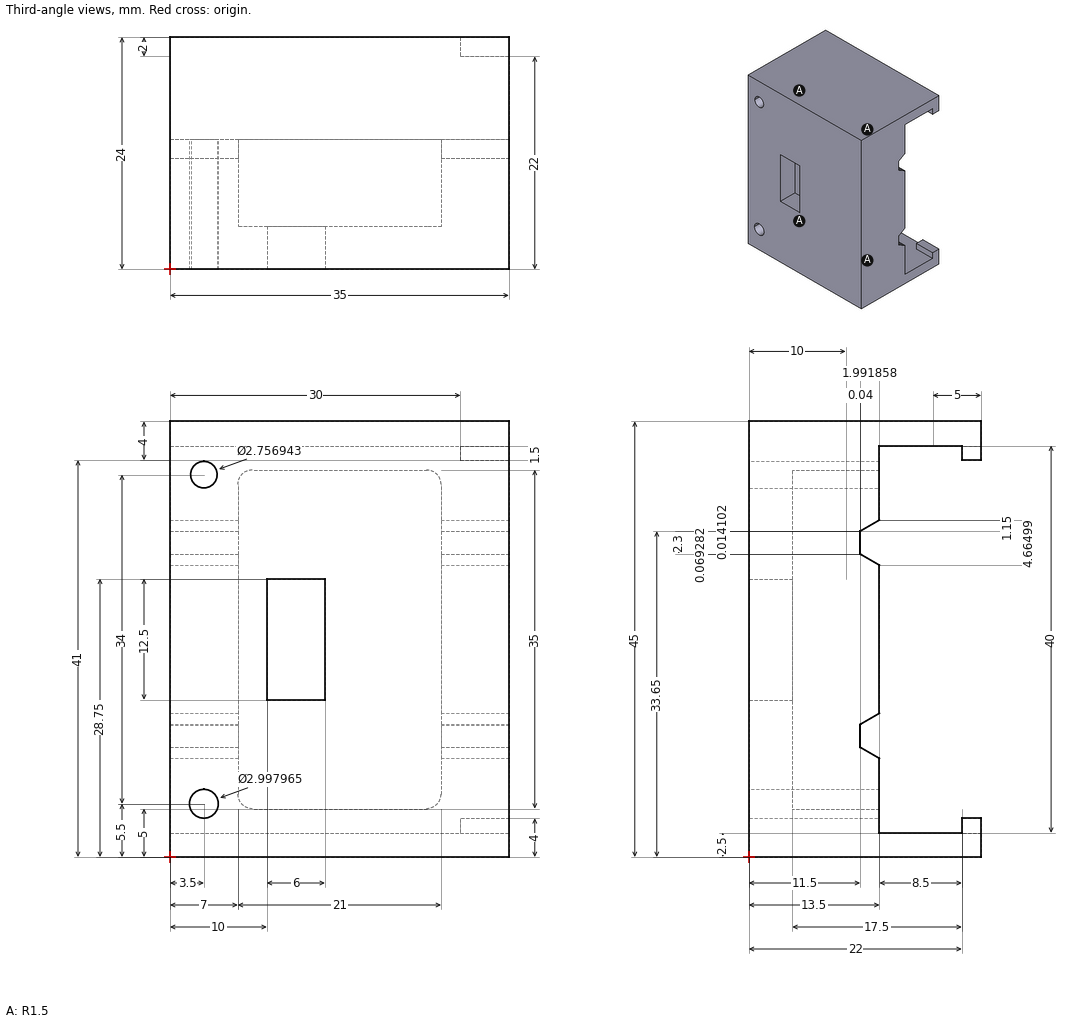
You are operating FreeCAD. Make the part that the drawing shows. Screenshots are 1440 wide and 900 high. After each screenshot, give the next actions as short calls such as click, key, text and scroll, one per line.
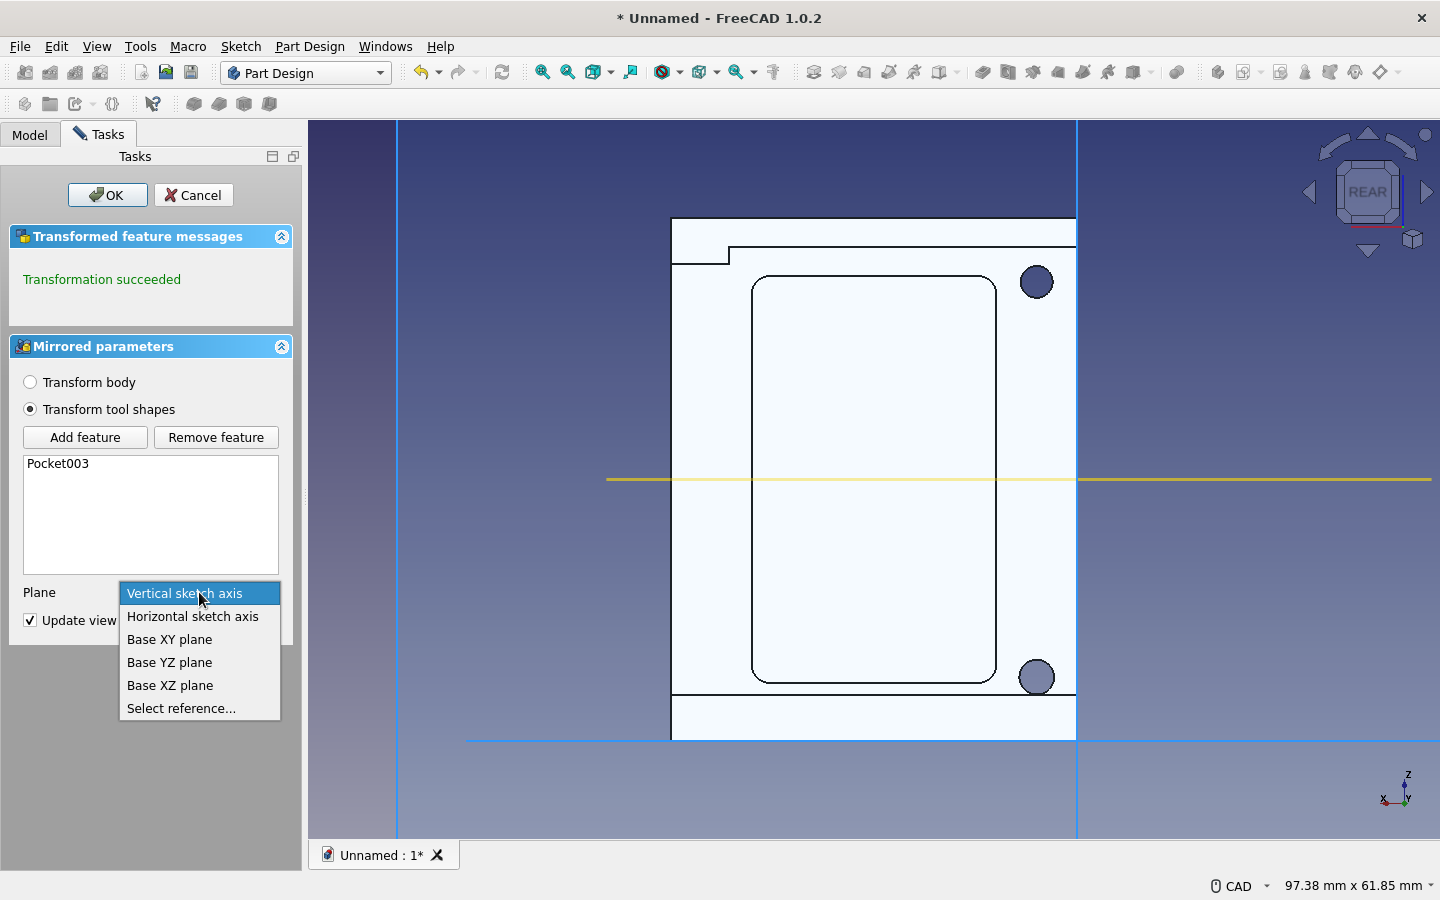
click(198, 708)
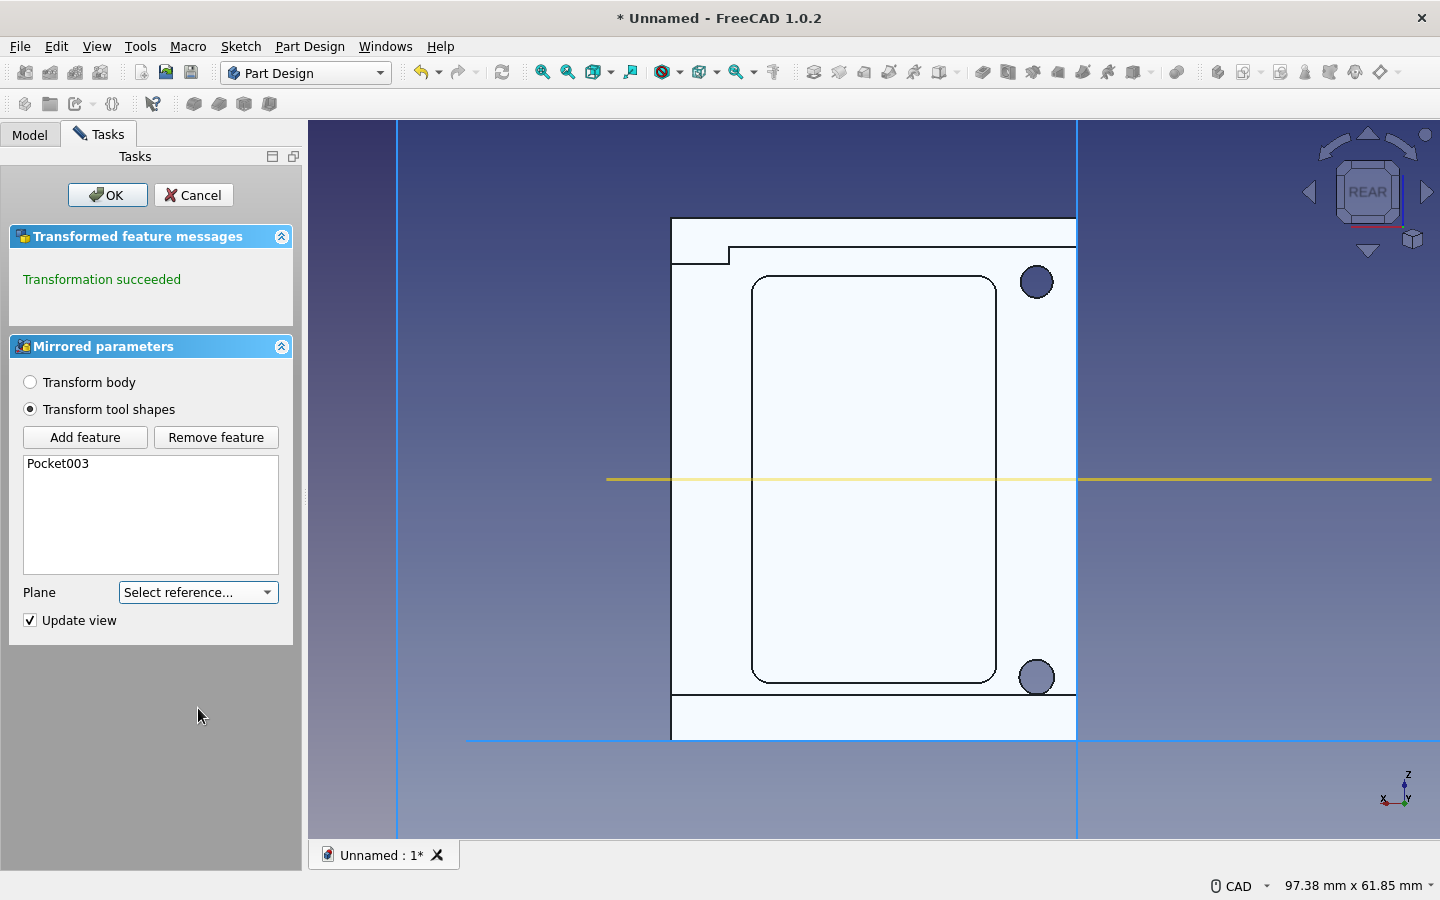
click(30, 134)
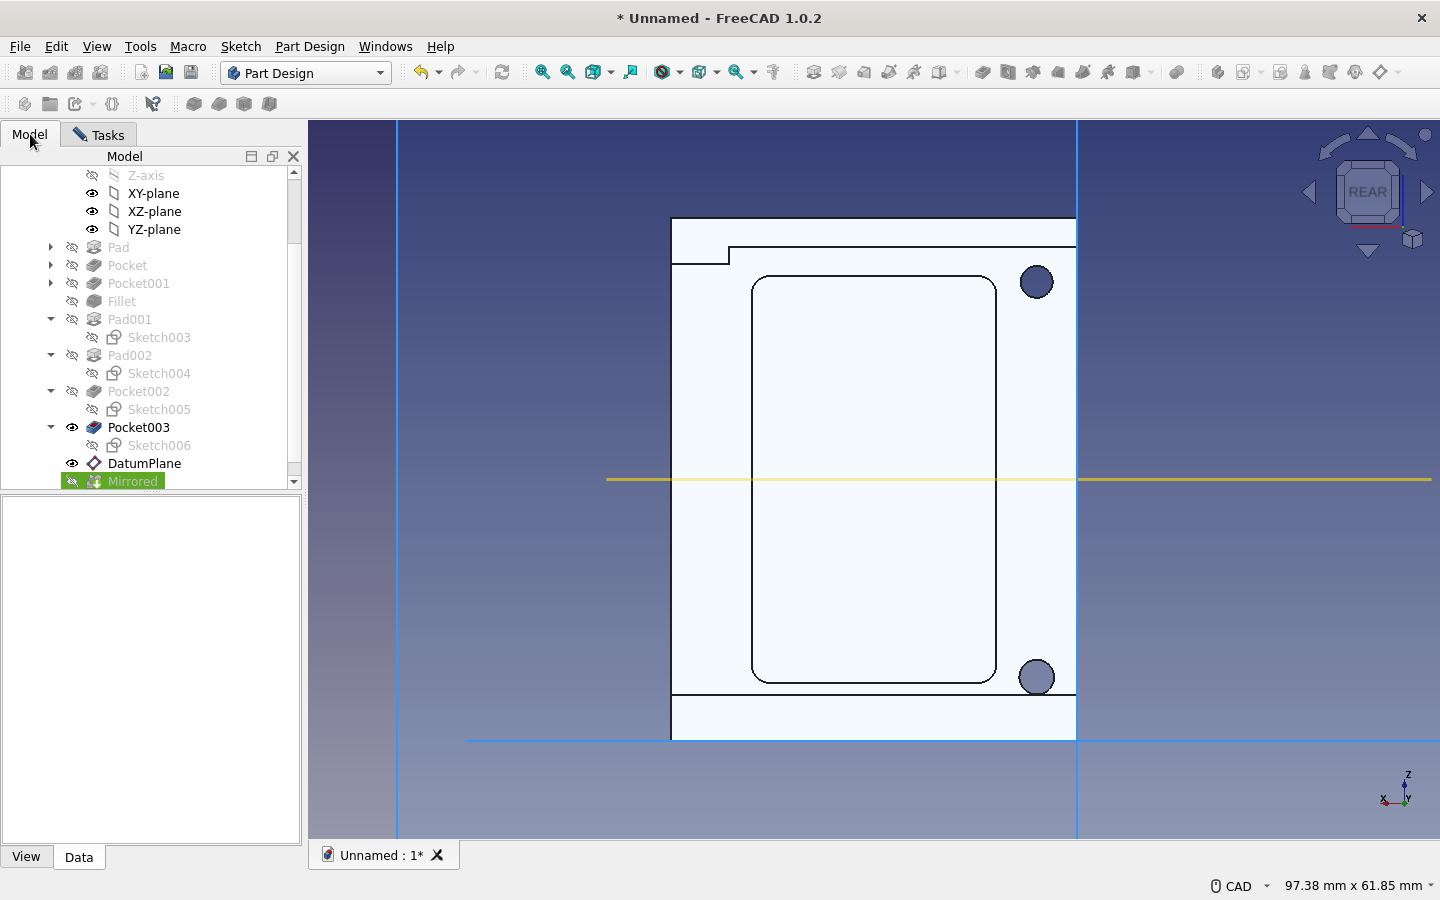
click(117, 463)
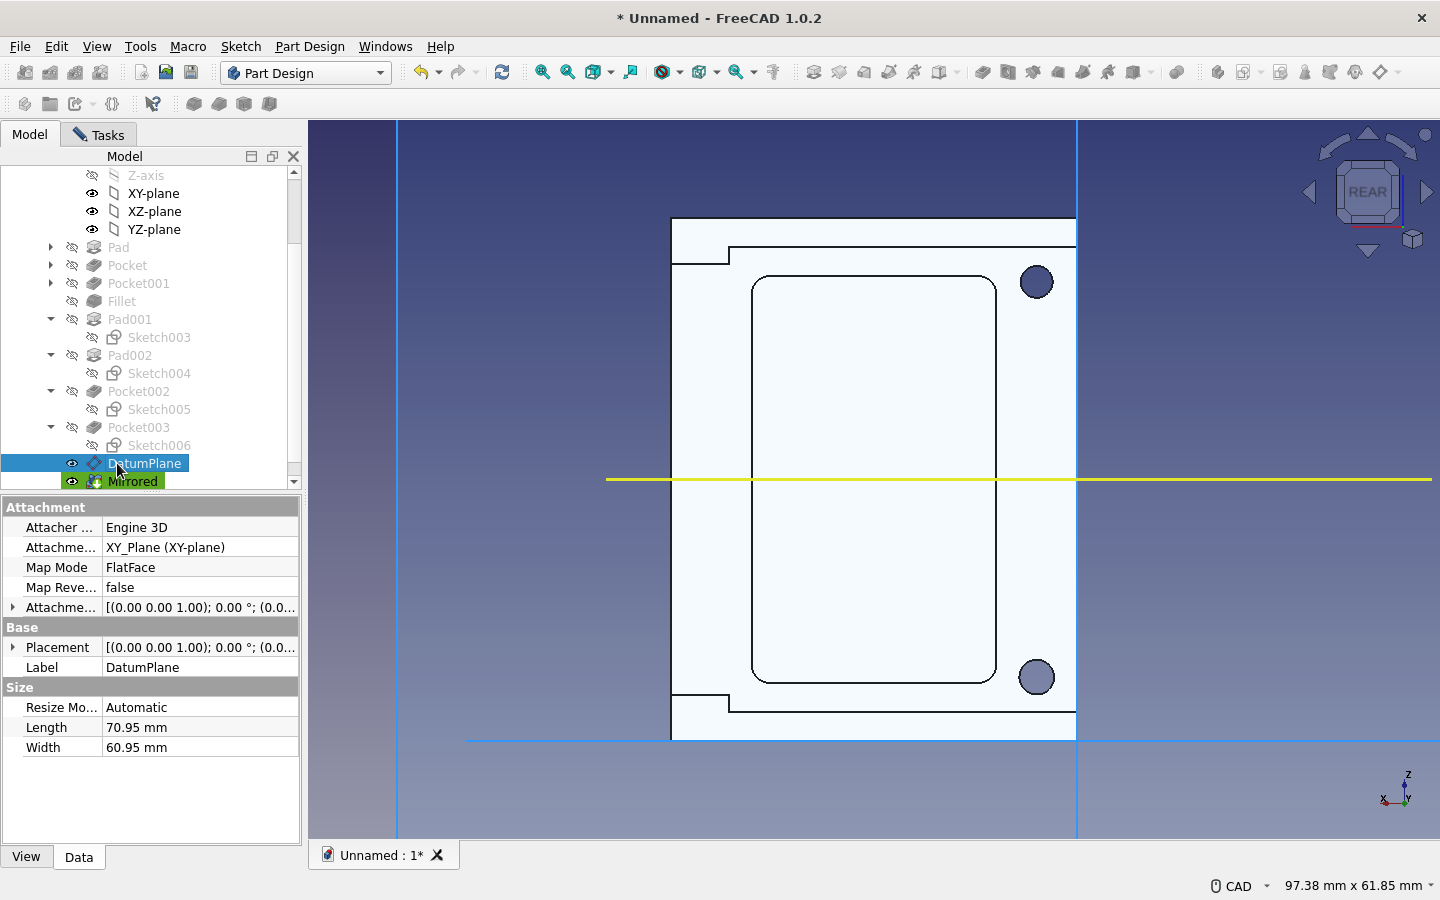
click(98, 134)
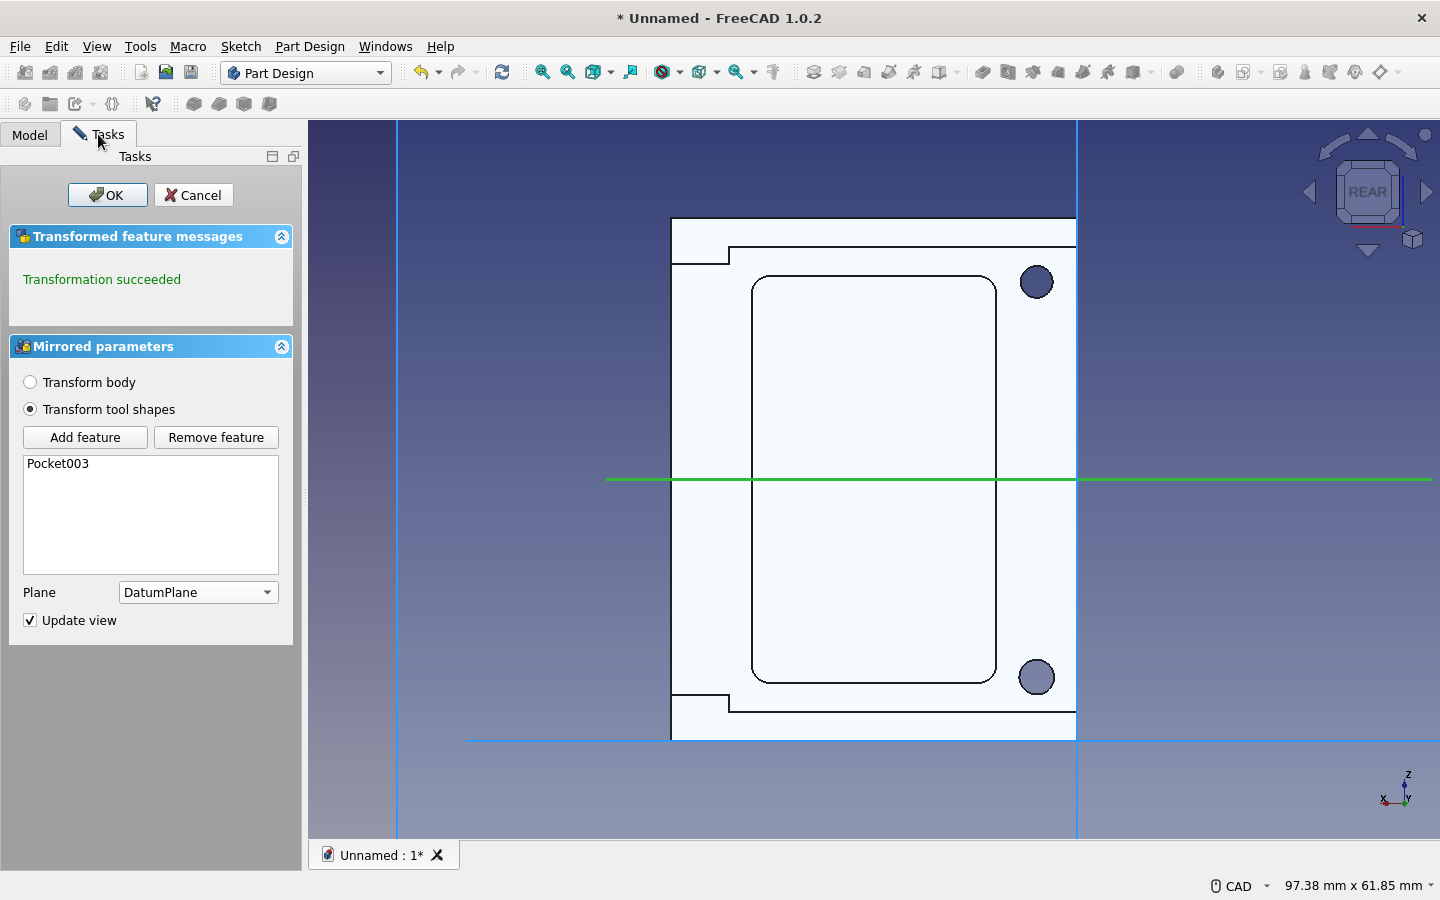
click(108, 195)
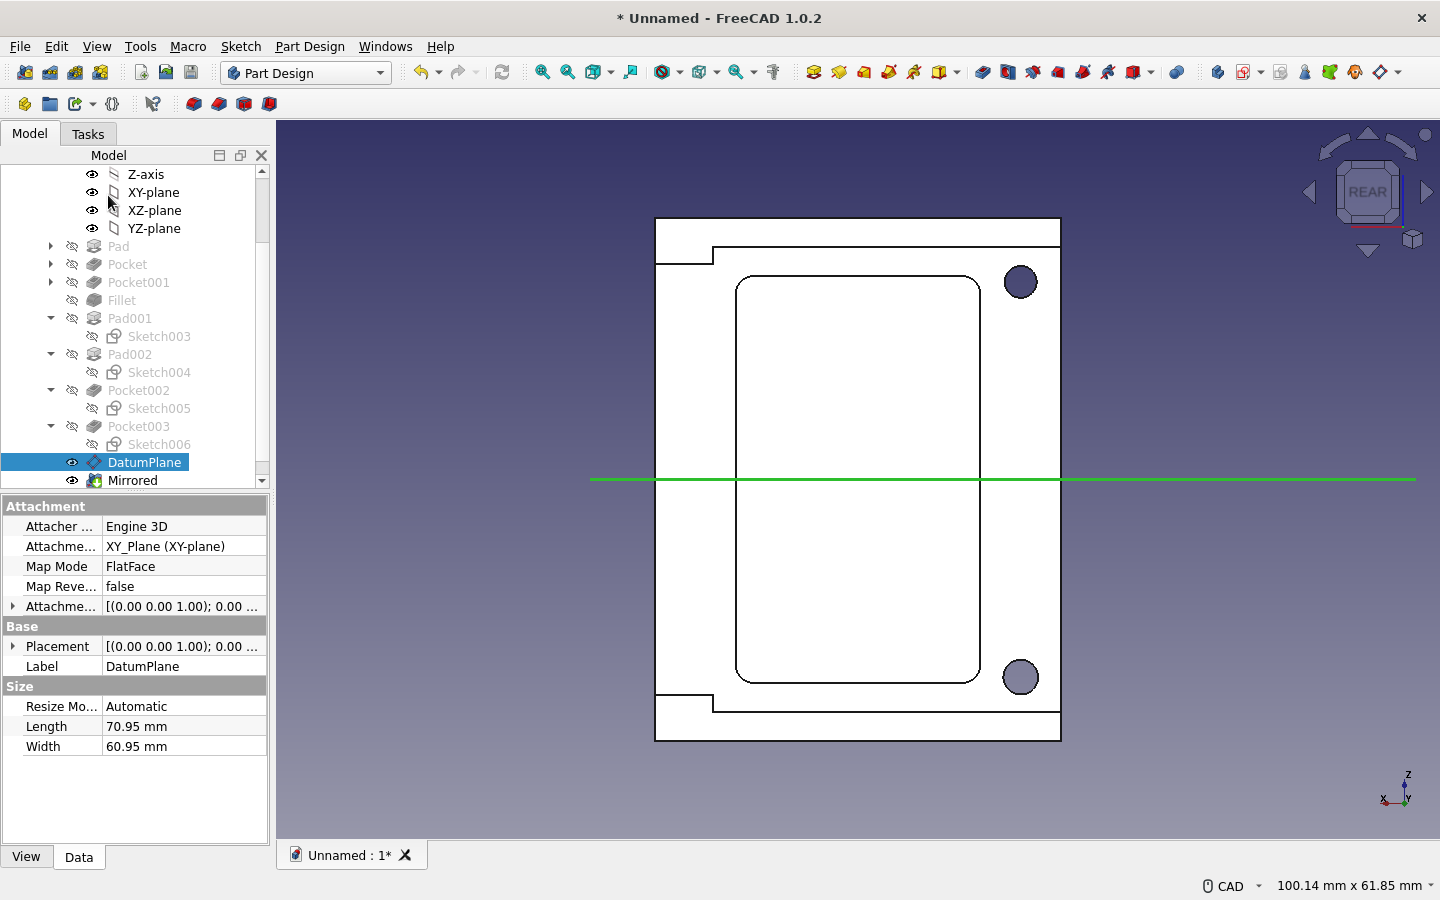
click(117, 462)
key(space)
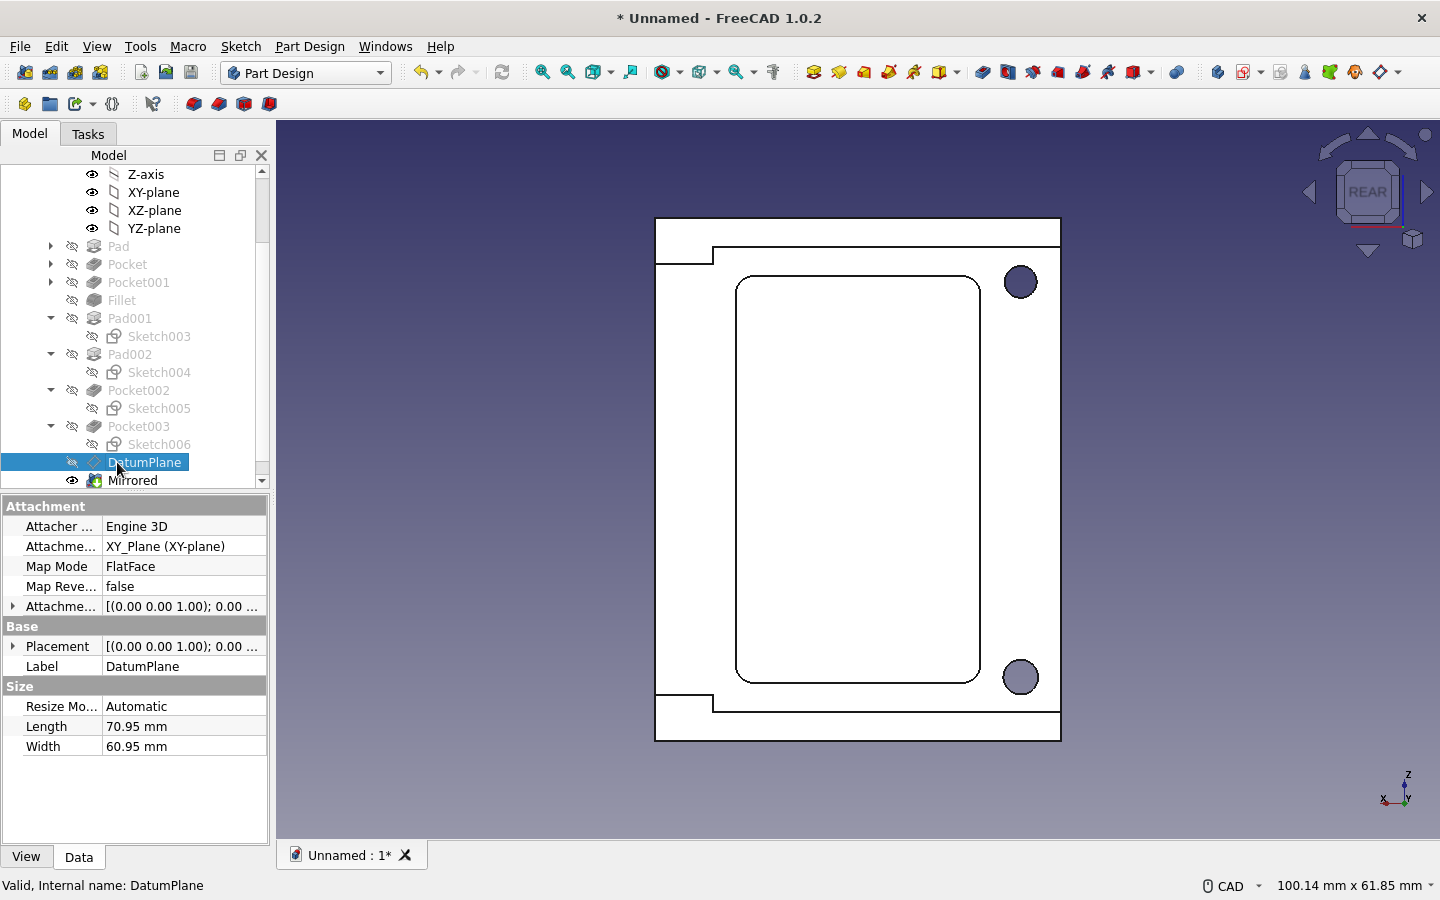
key(0)